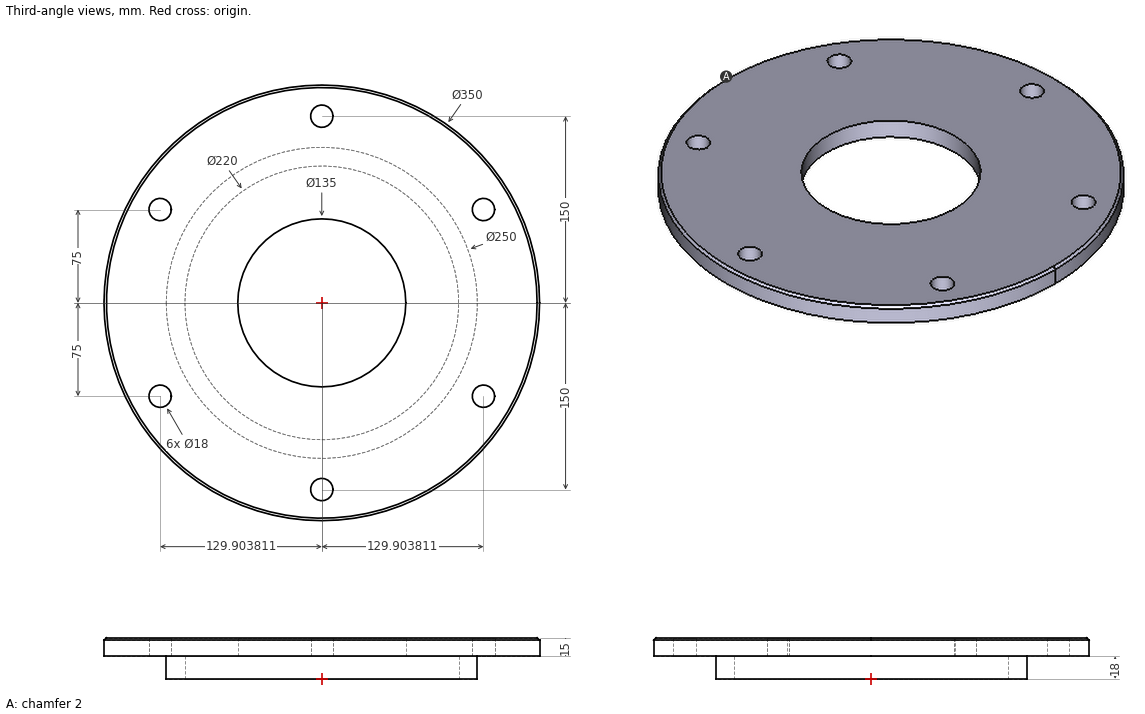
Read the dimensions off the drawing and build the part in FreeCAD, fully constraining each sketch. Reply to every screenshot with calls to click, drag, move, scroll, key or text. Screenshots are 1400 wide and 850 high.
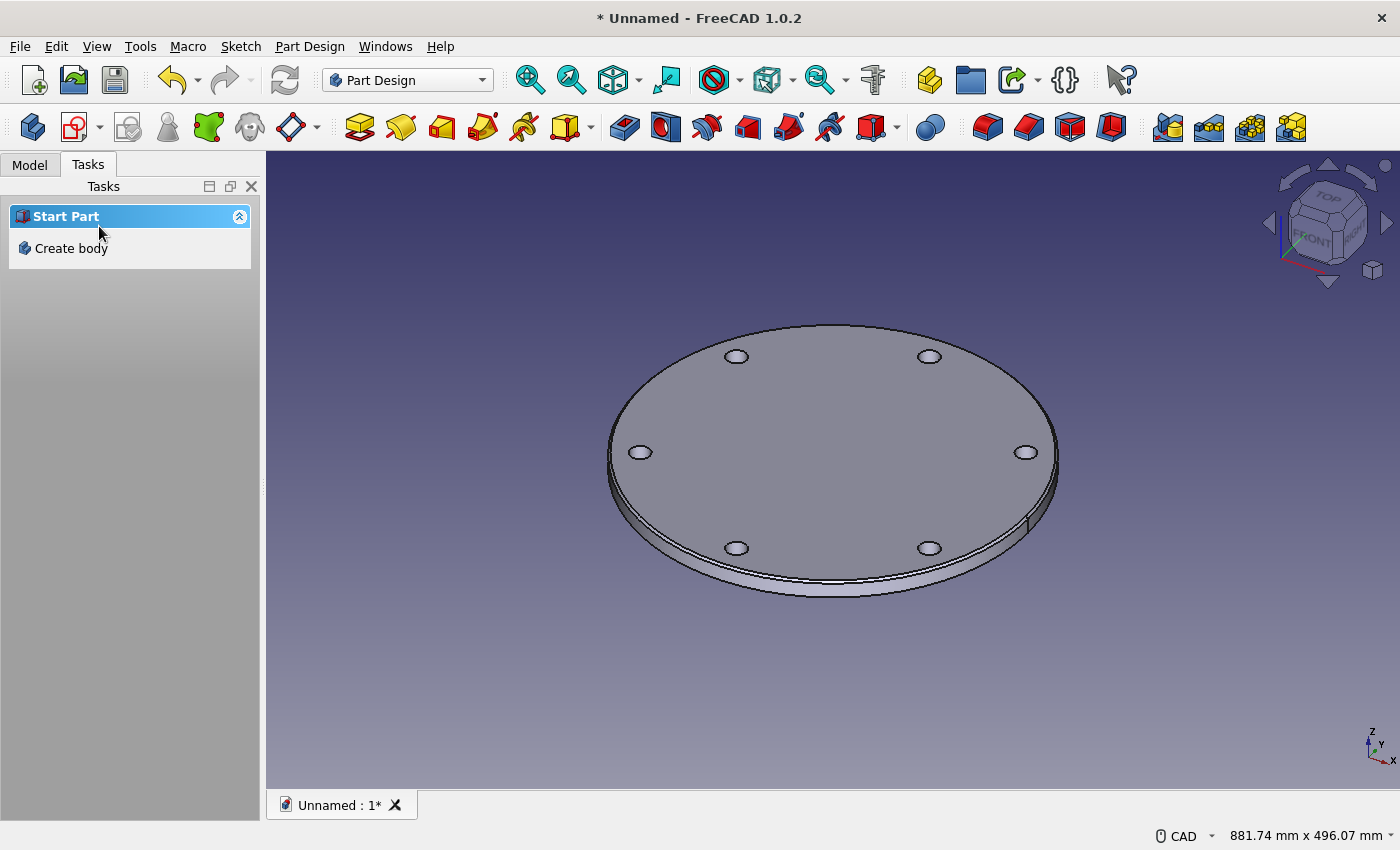
click(833, 452)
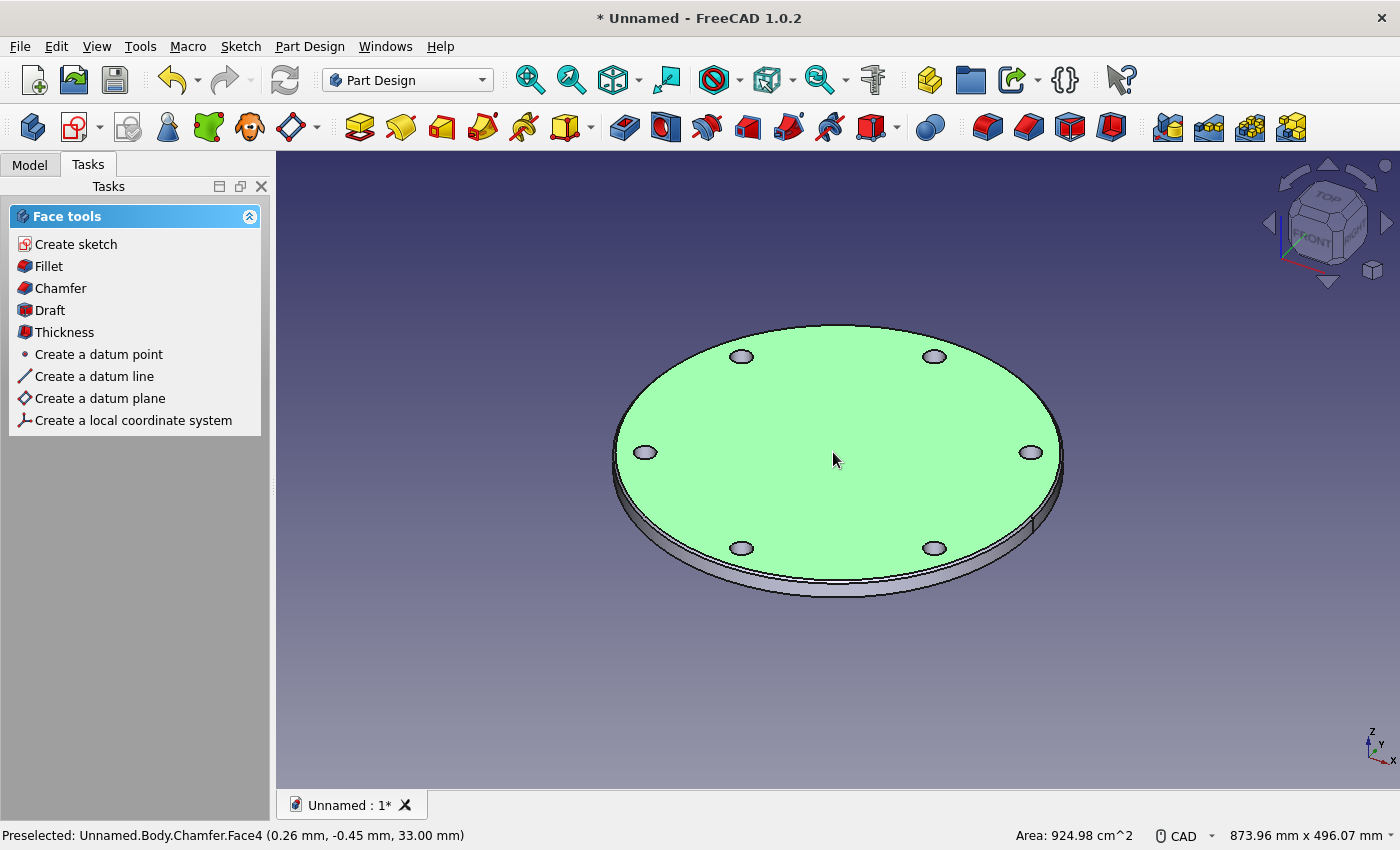
click(74, 128)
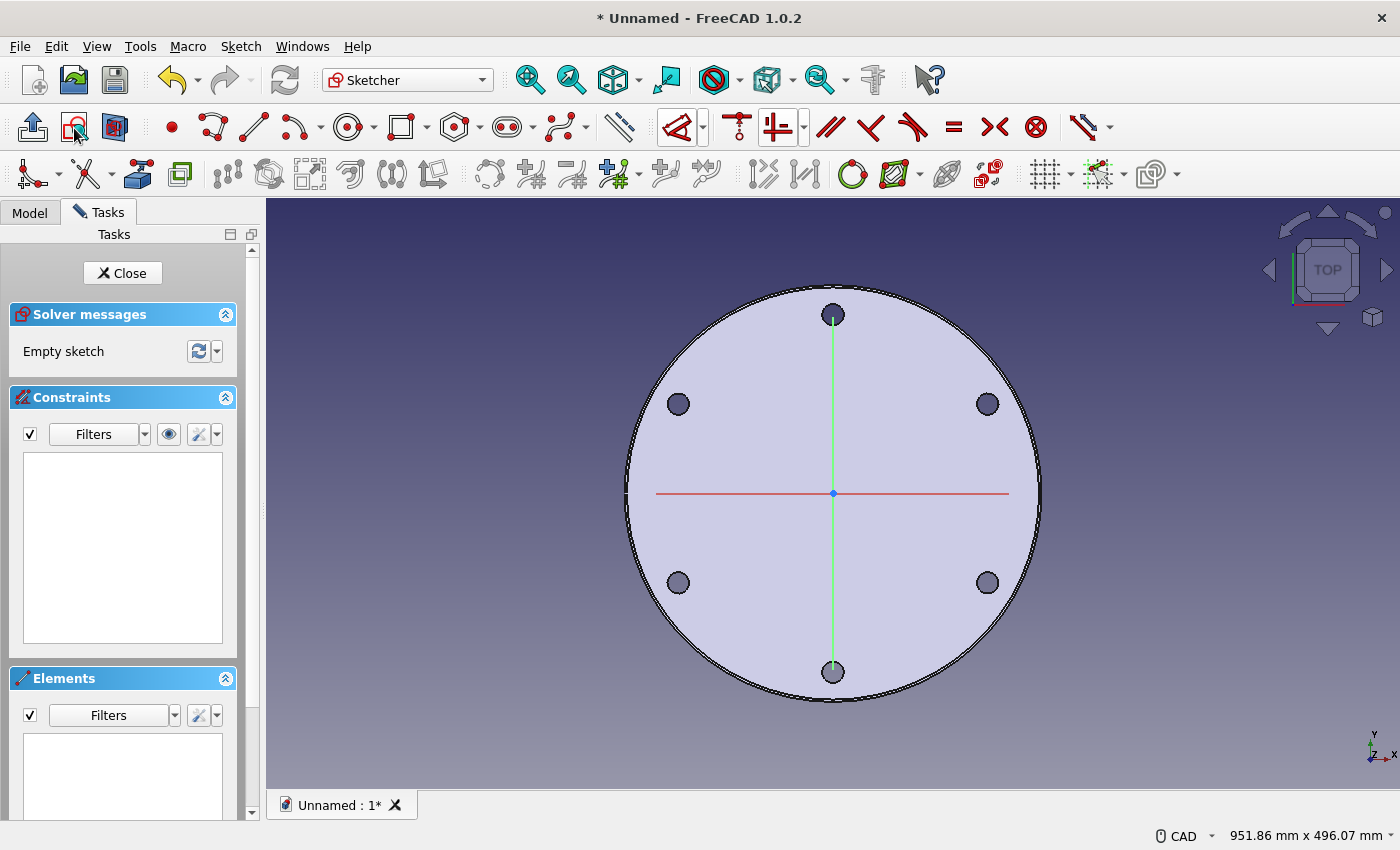
scroll(889, 494, up, 4)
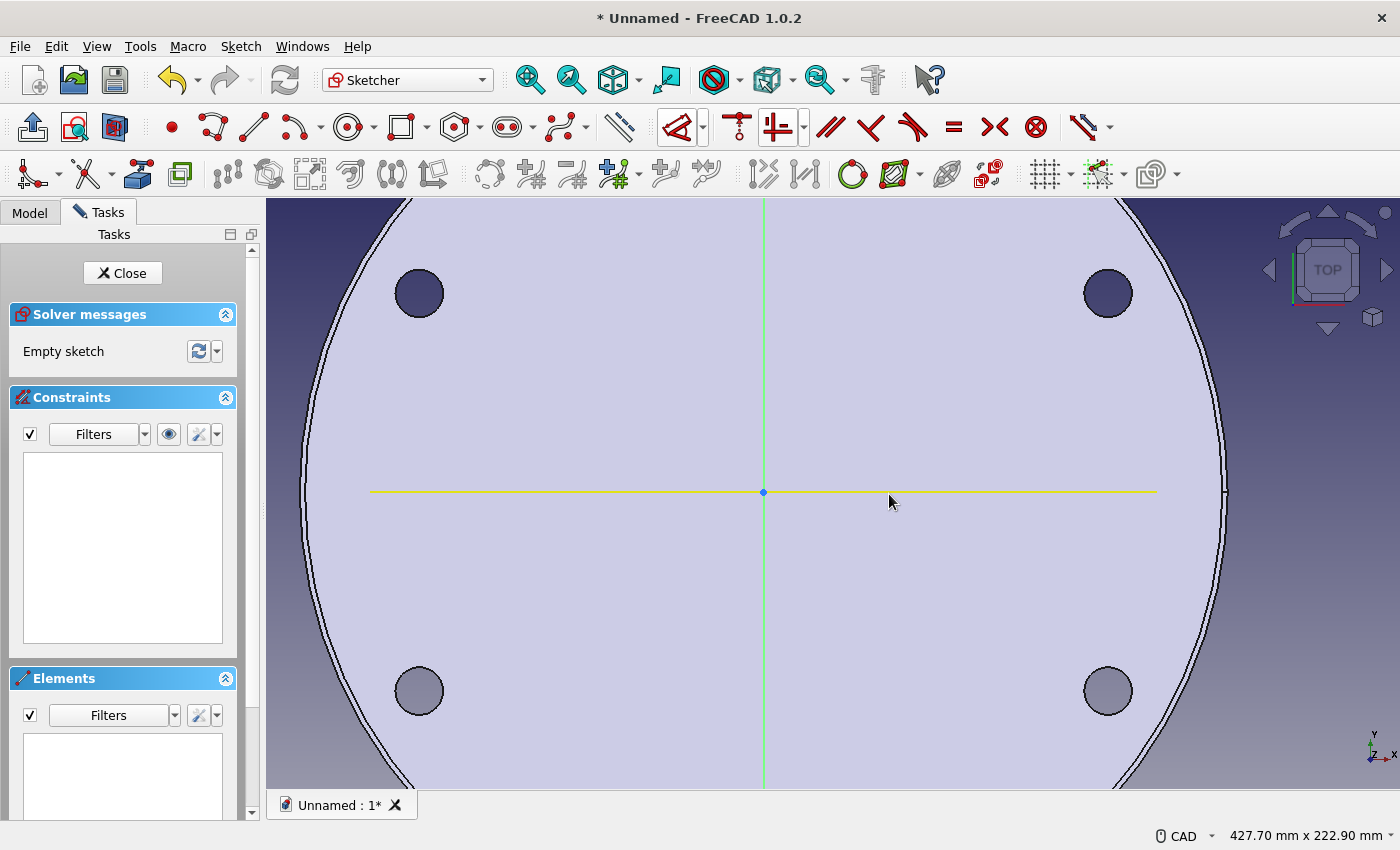
click(348, 128)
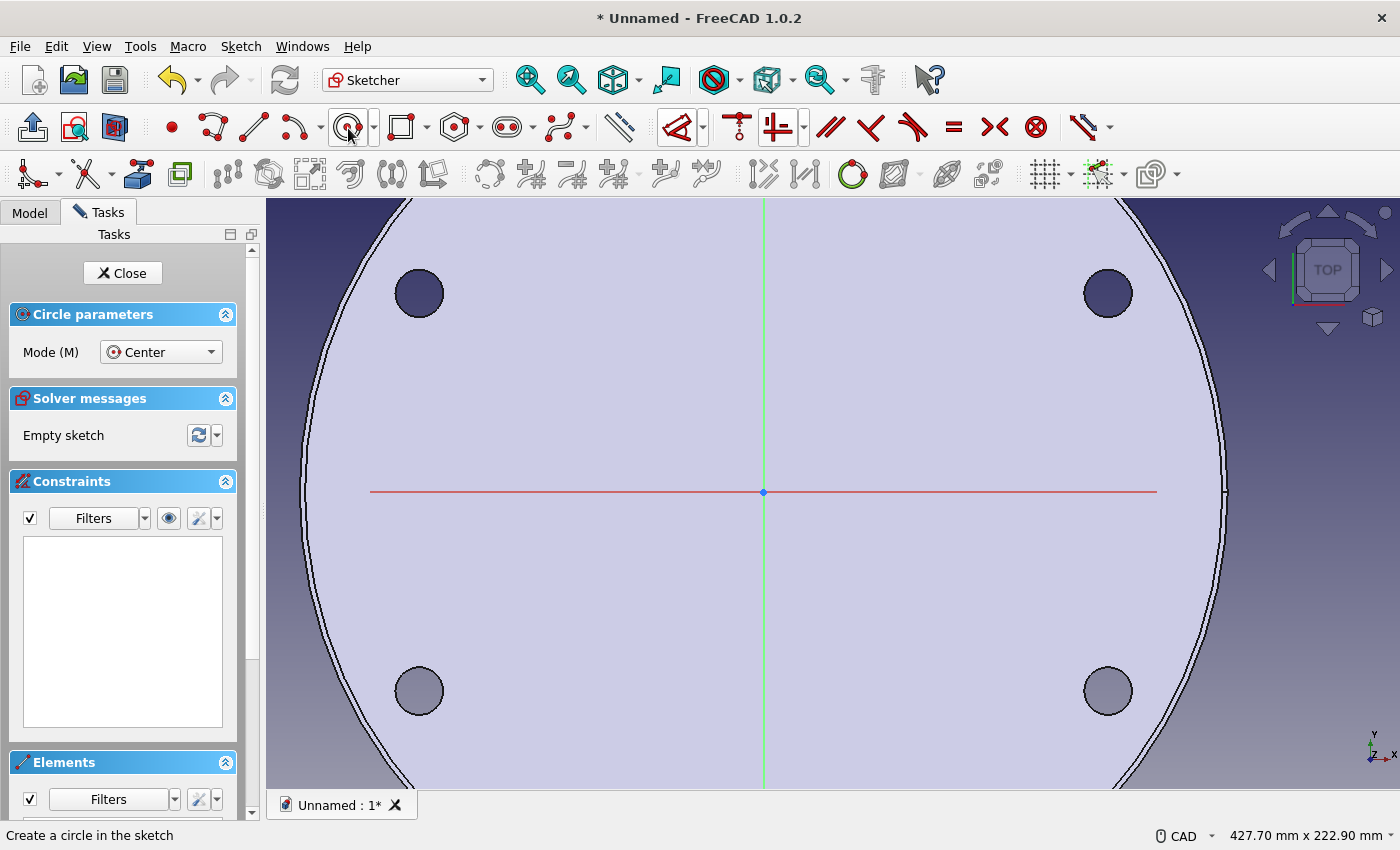
click(764, 492)
click(890, 366)
key(Escape)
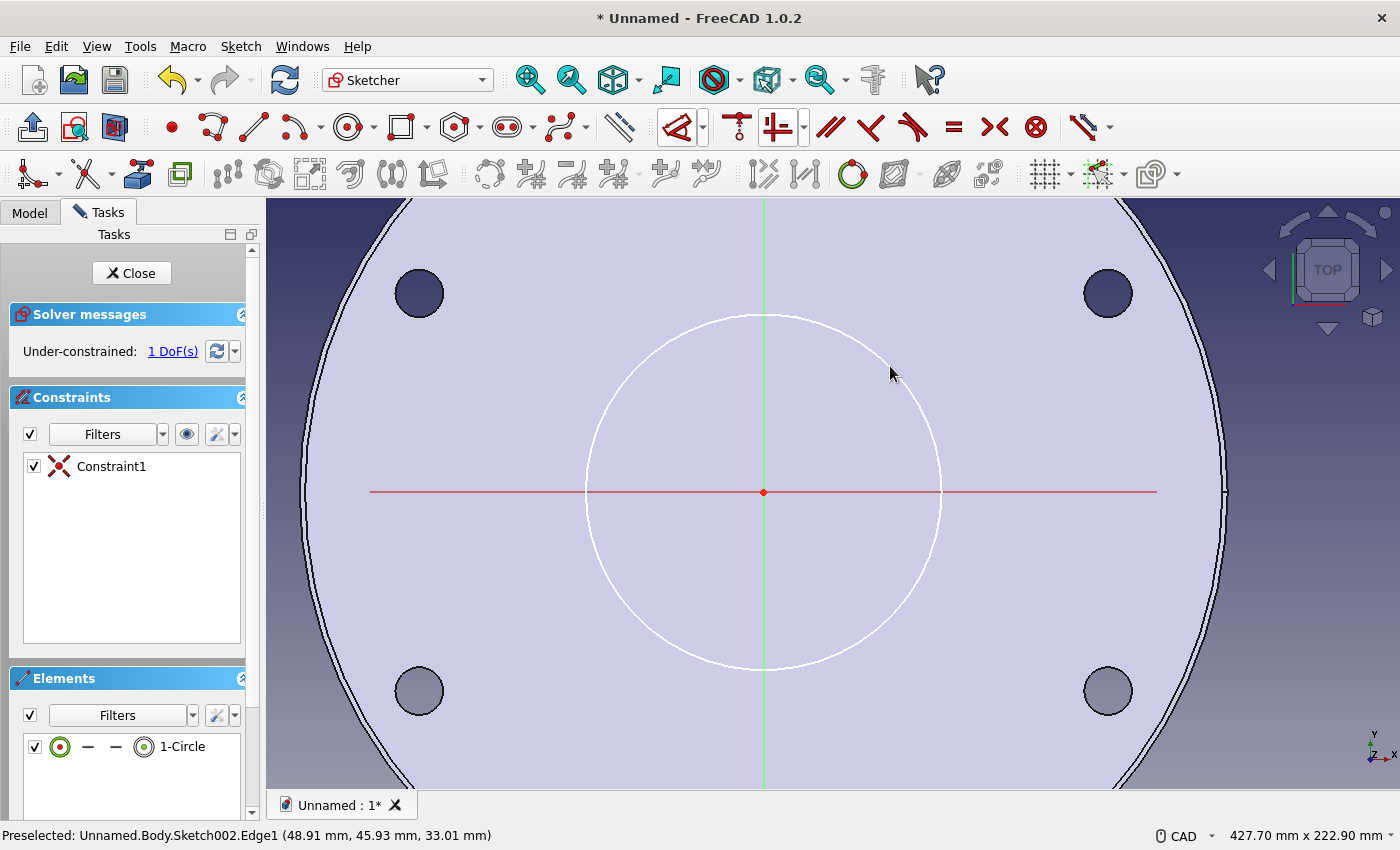
click(889, 366)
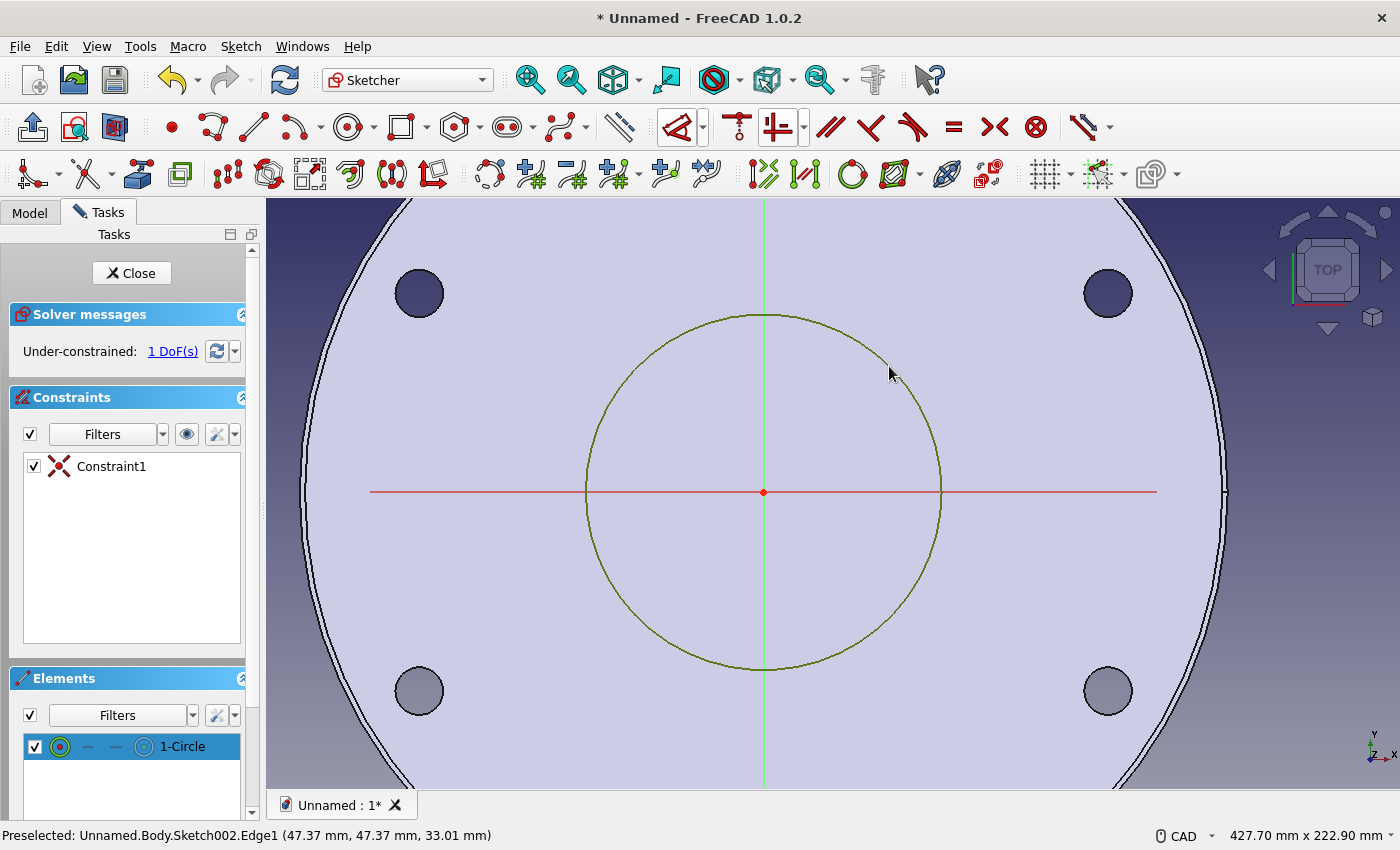
key(k)
key(o)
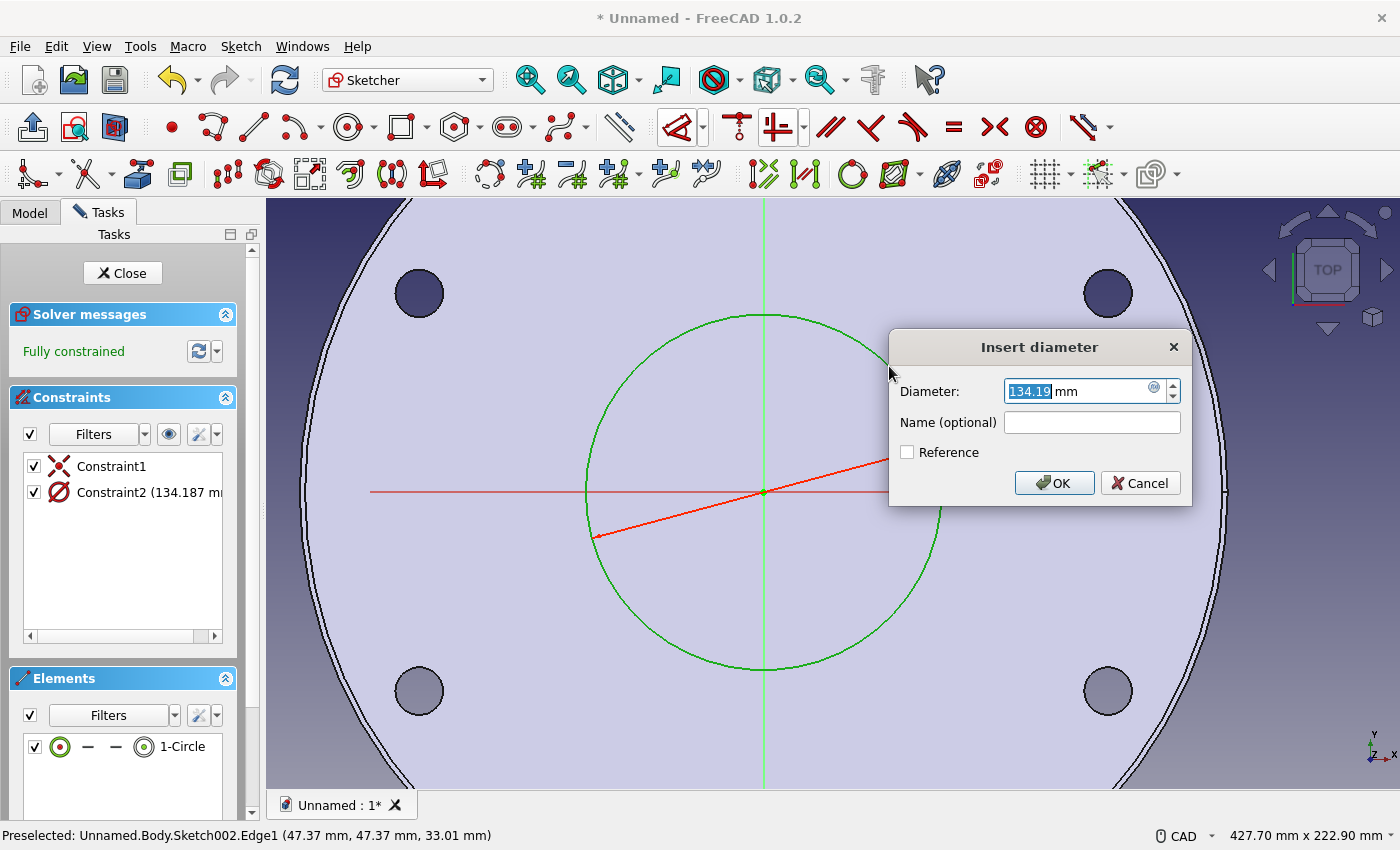
text(135)
key(Return)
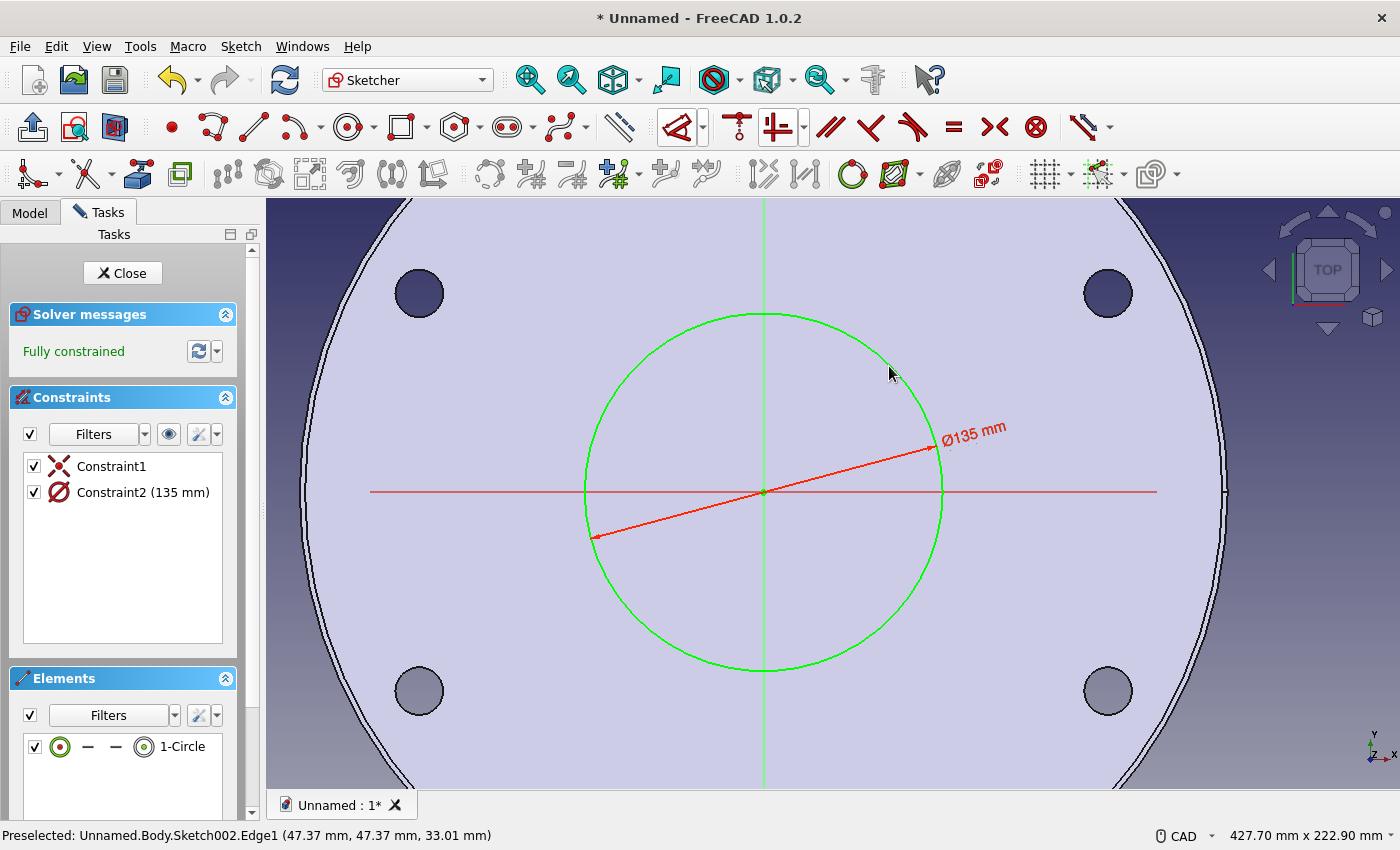
click(123, 273)